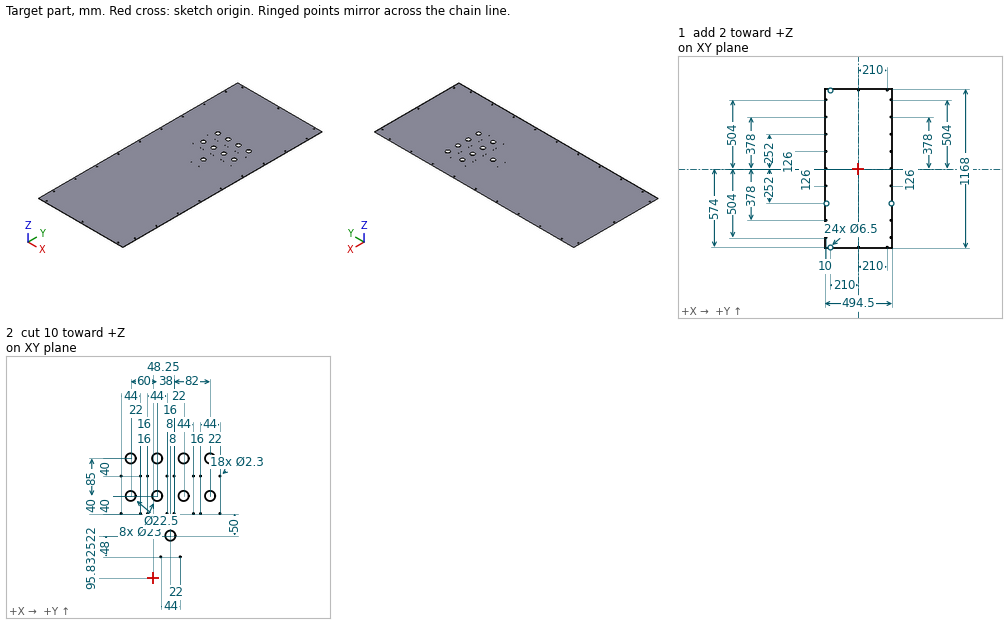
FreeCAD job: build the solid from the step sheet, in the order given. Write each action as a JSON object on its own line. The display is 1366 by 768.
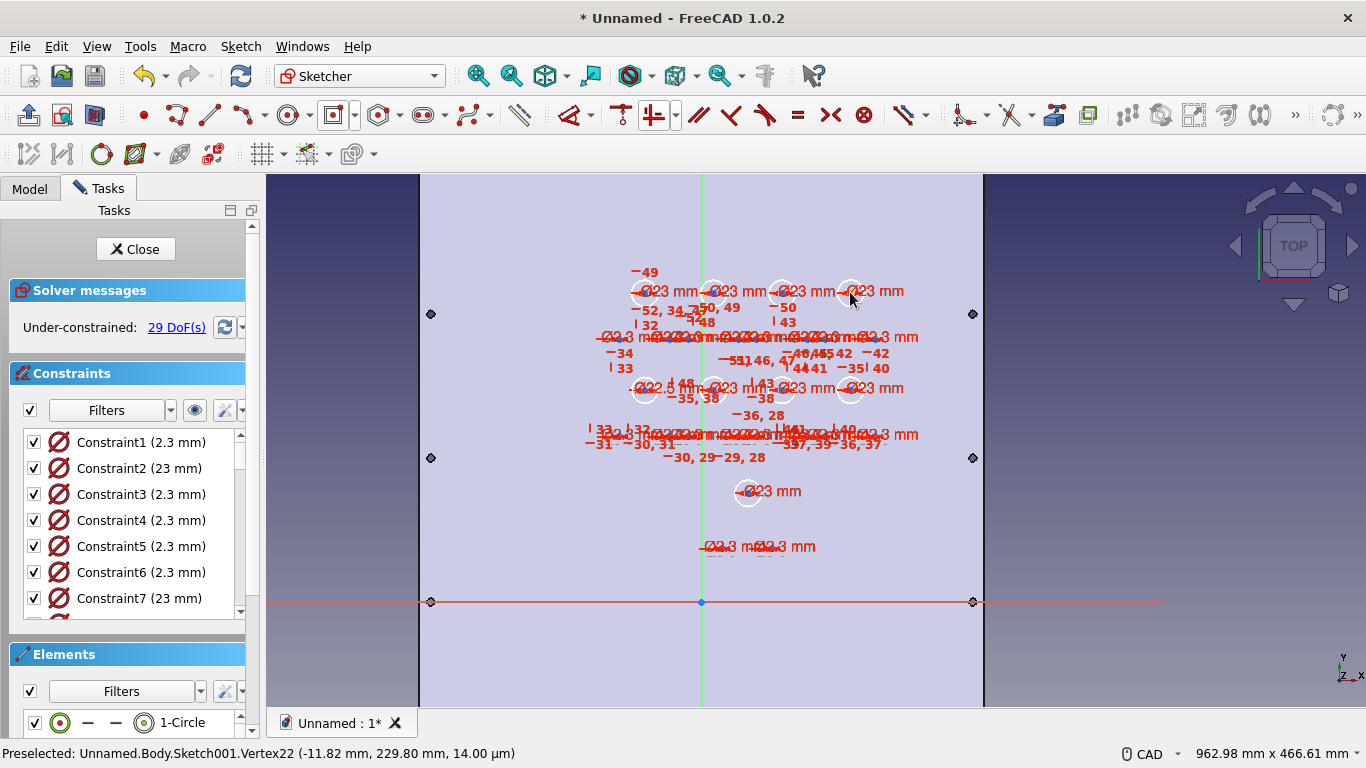
{"action": "left_click", "coordinate": [773, 549]}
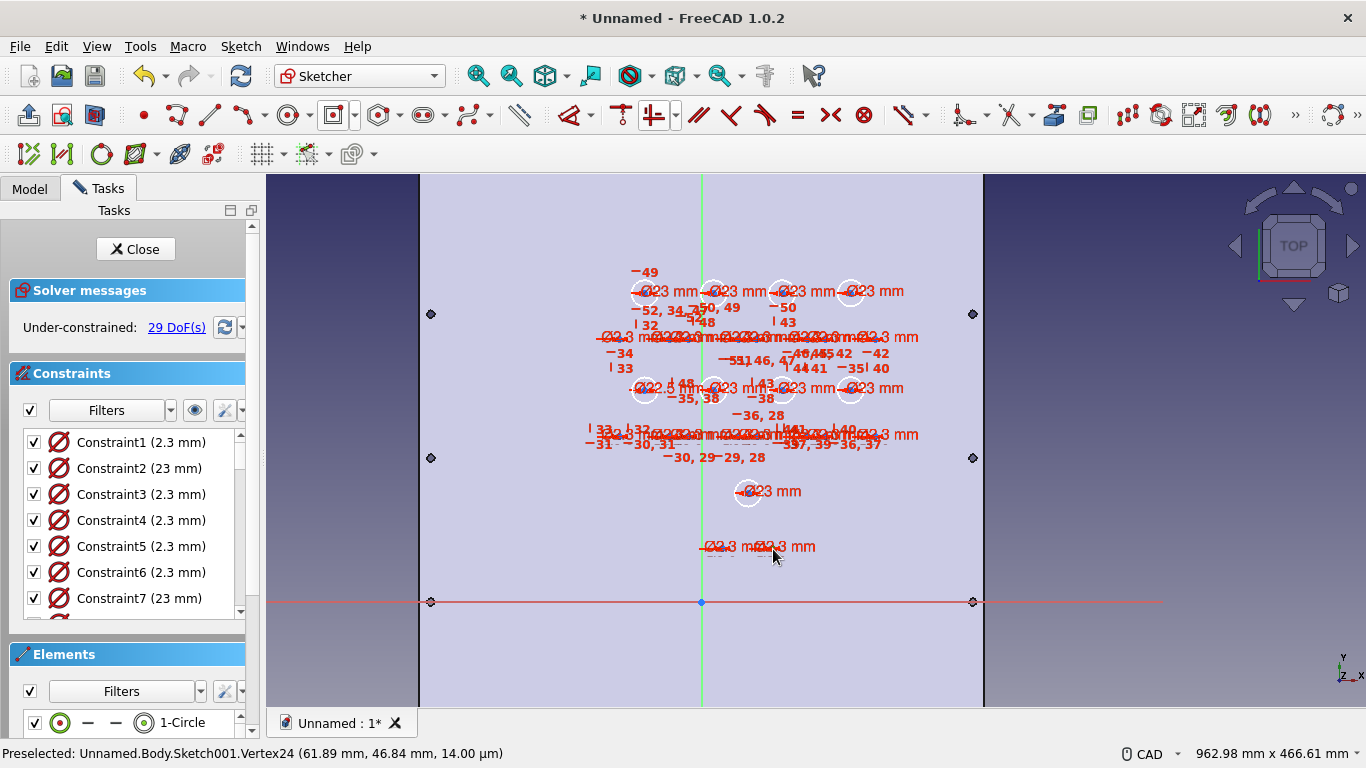
{"action": "left_click", "coordinate": [723, 549]}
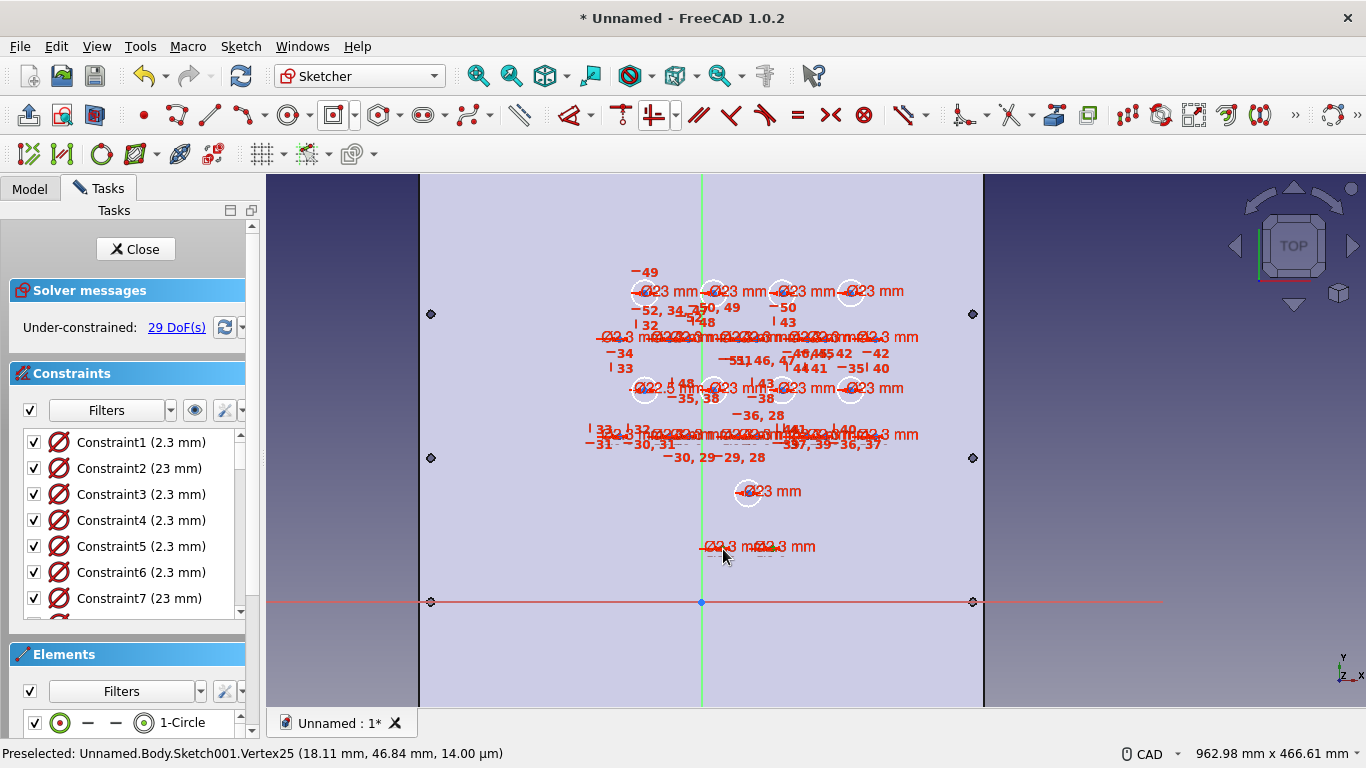
{"action": "key", "text": "h"}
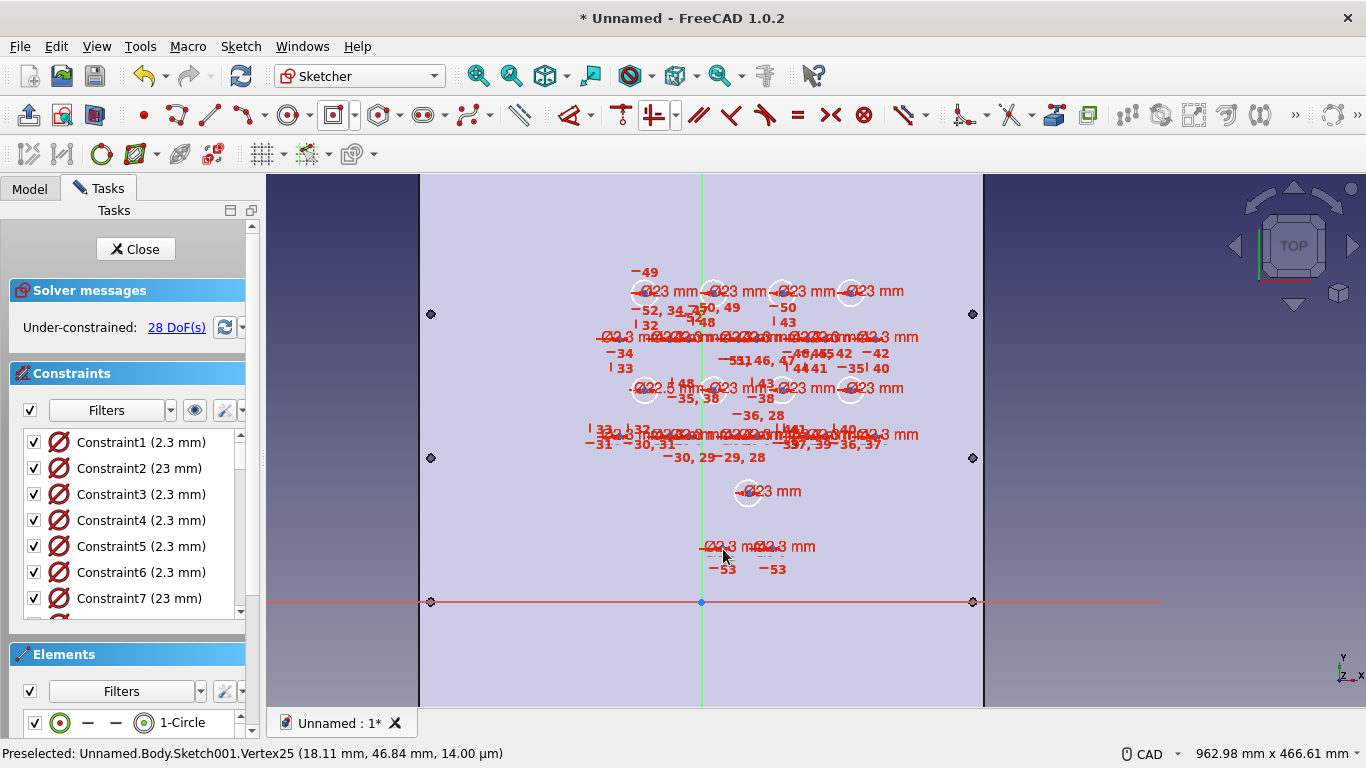
{"action": "left_click", "coordinate": [851, 390]}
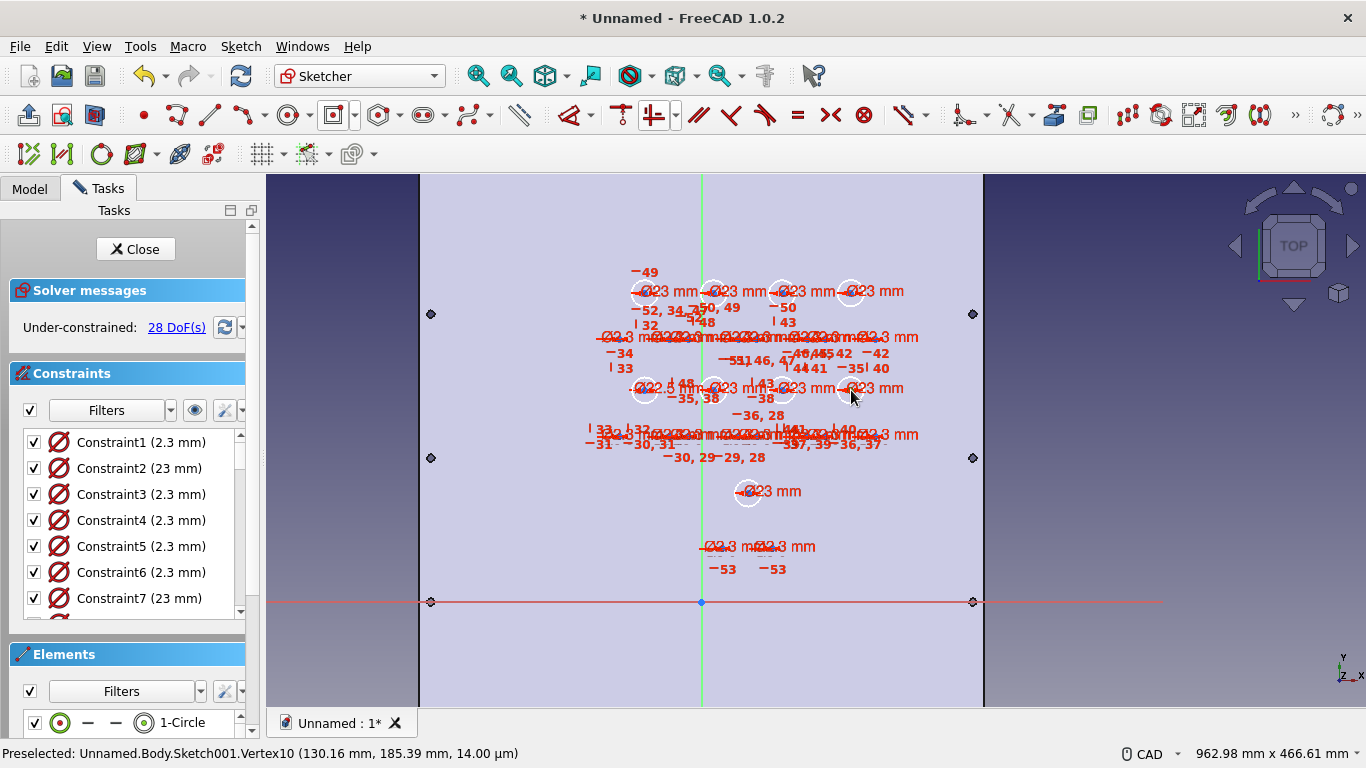
{"action": "left_click", "coordinate": [851, 293]}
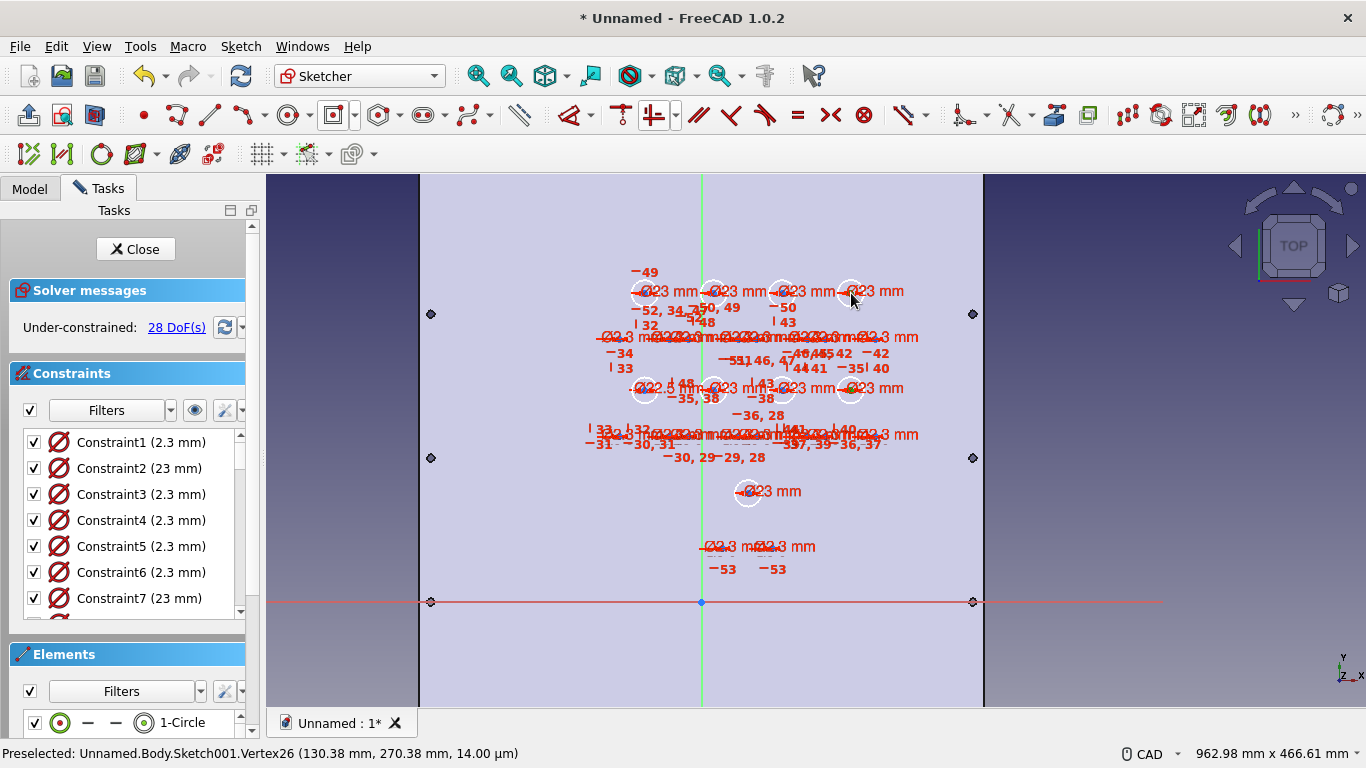
{"action": "key", "text": "v"}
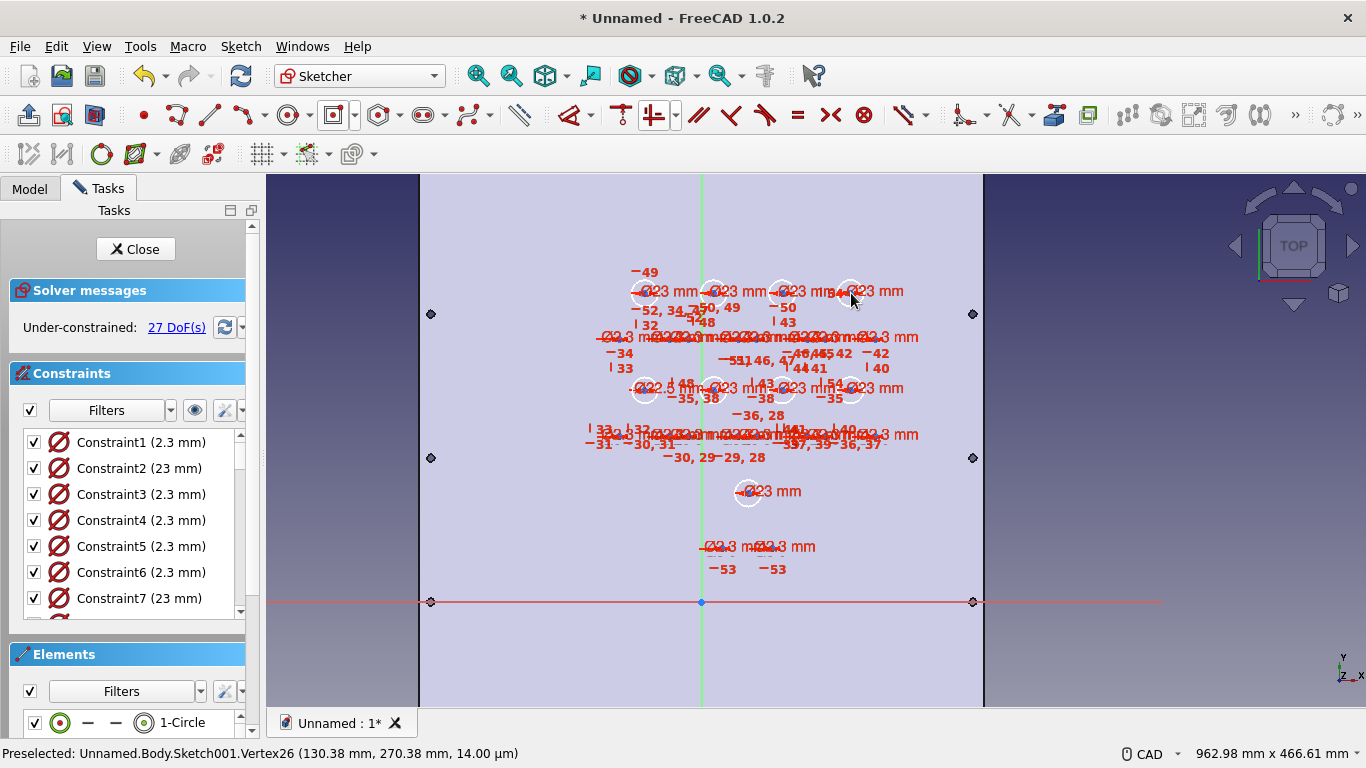
{"action": "left_click", "coordinate": [782, 293]}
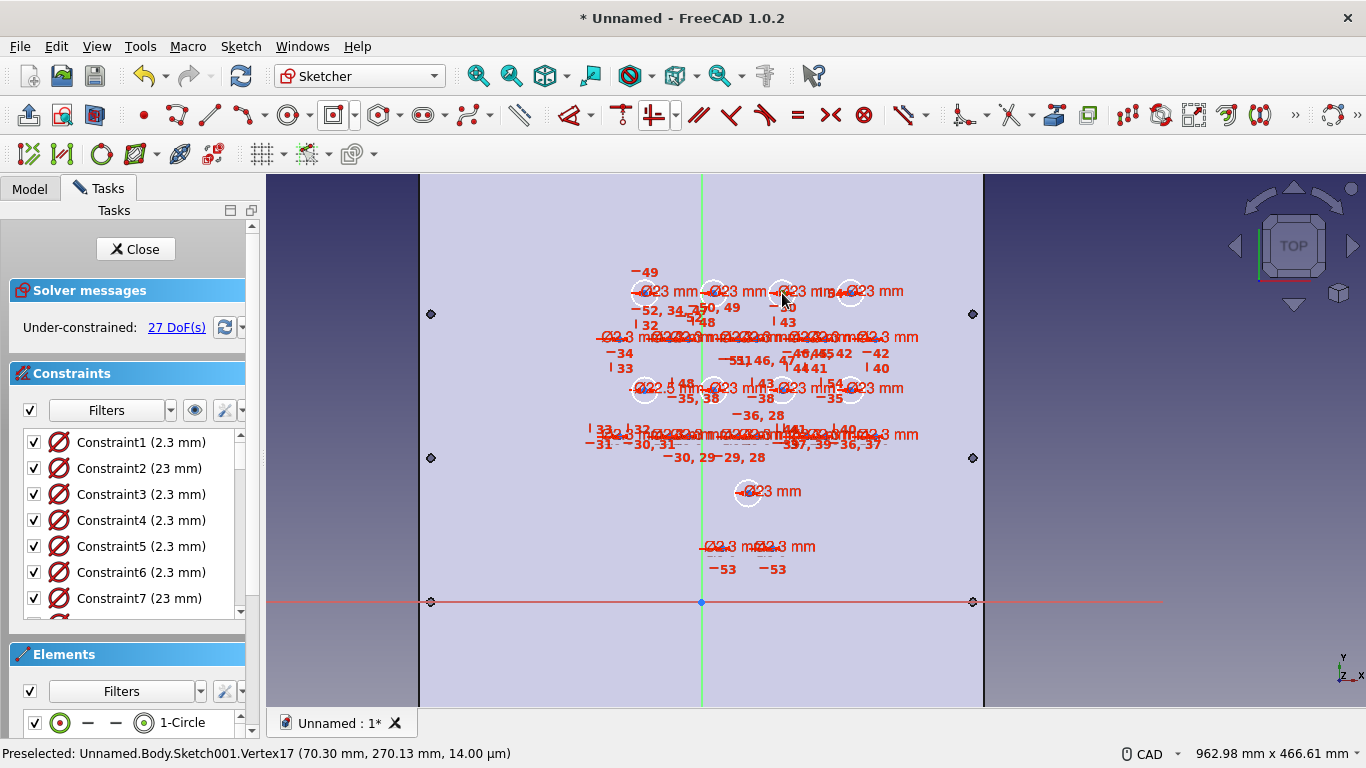
{"action": "left_click", "coordinate": [851, 293]}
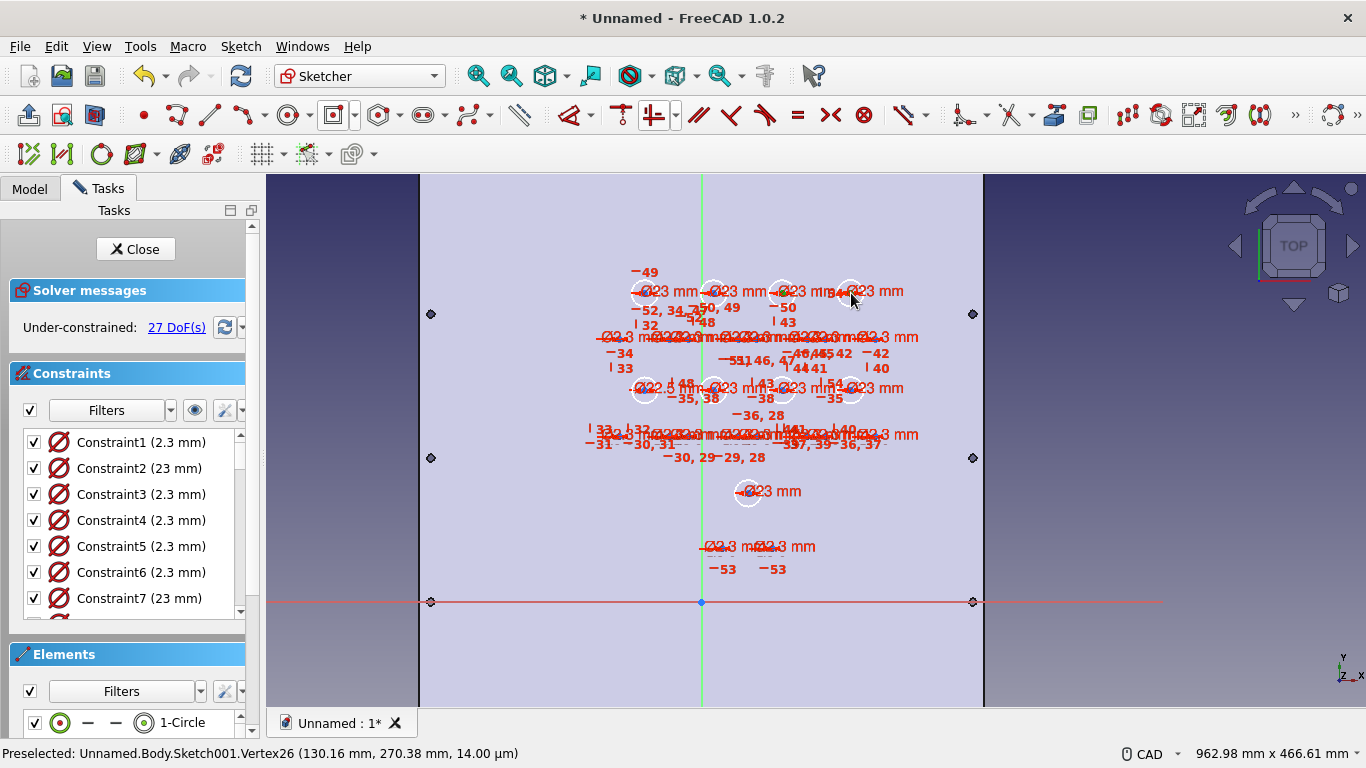
{"action": "left_click", "coordinate": [676, 116]}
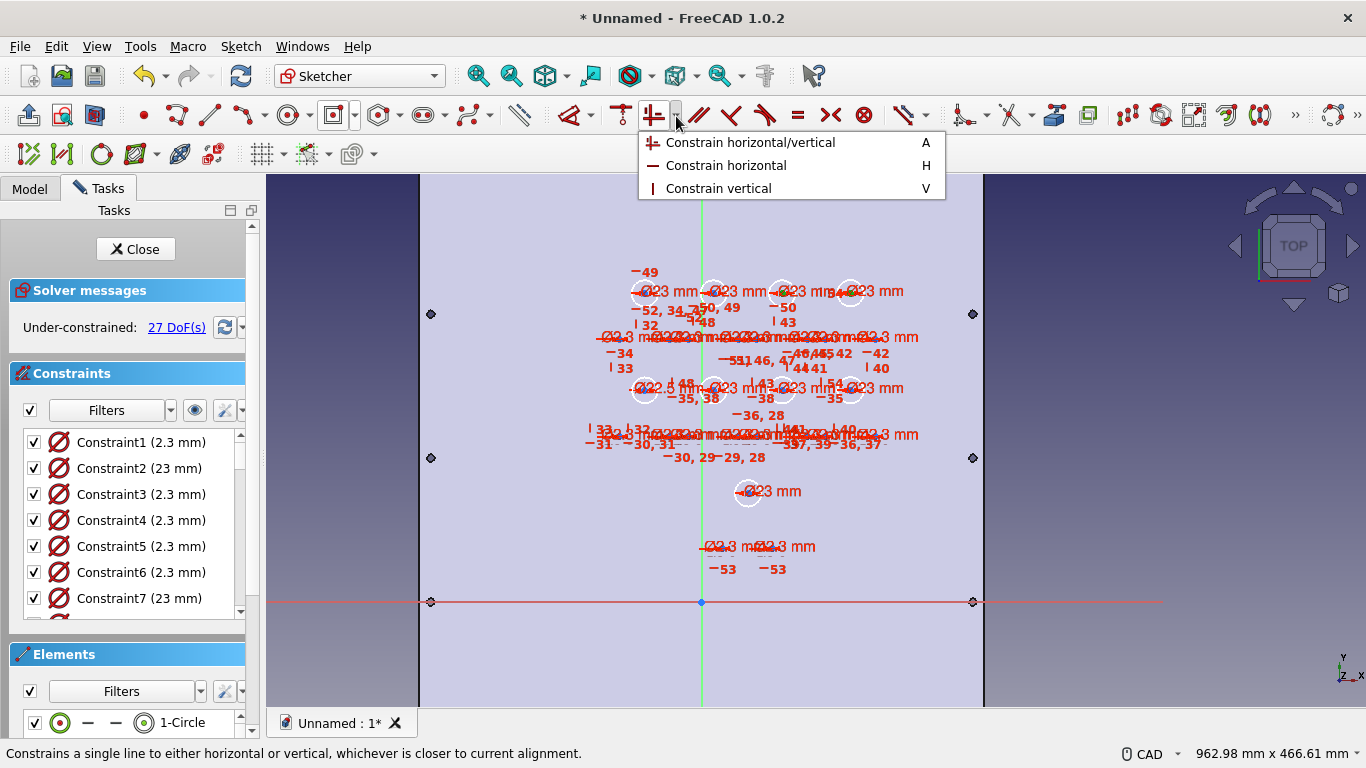
{"action": "left_click", "coordinate": [792, 166]}